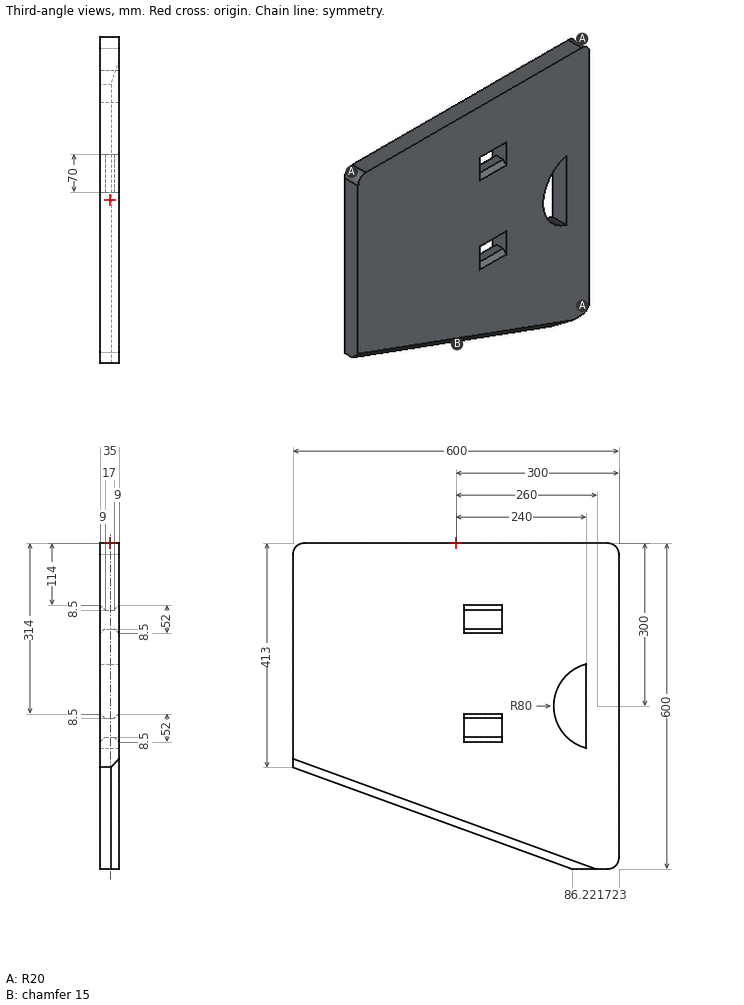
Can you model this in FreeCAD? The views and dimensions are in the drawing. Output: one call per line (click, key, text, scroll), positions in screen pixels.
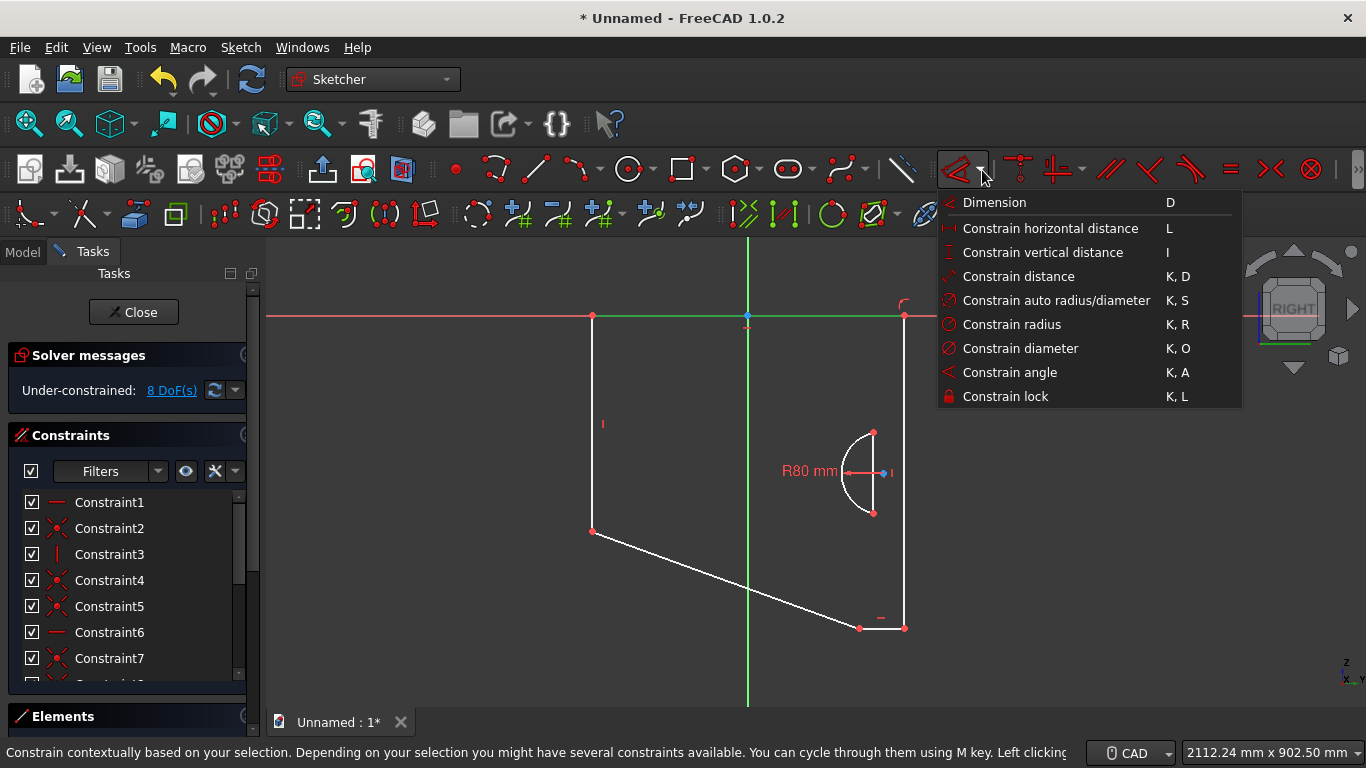
click(1090, 228)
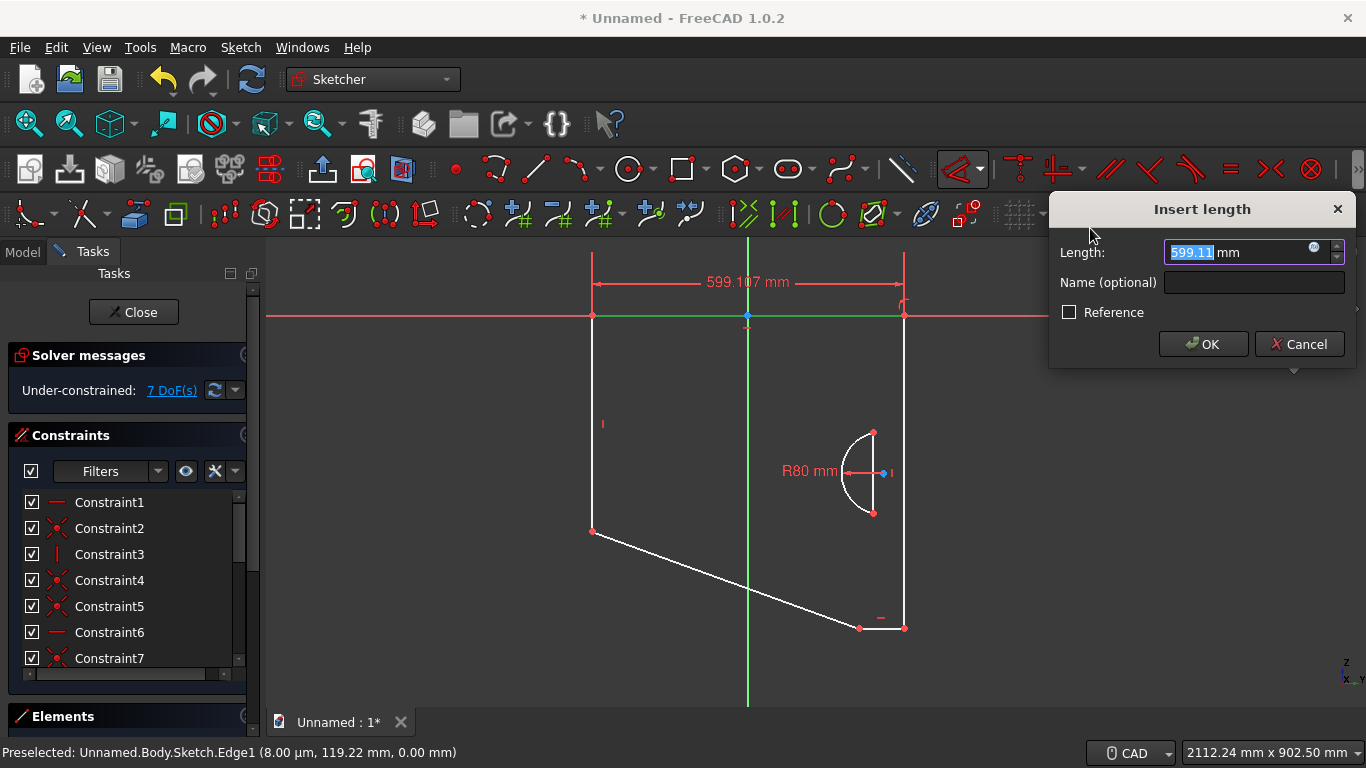
text(600)
key(Return)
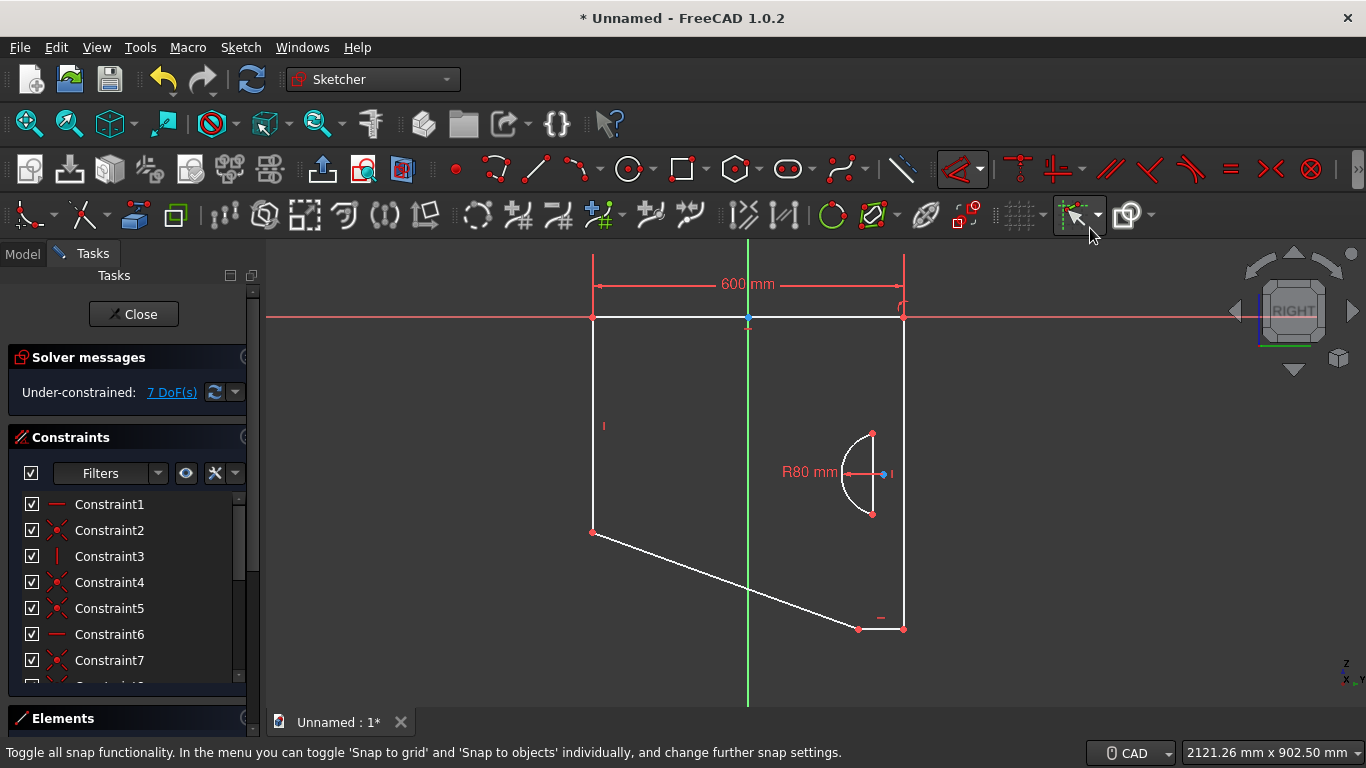
click(593, 382)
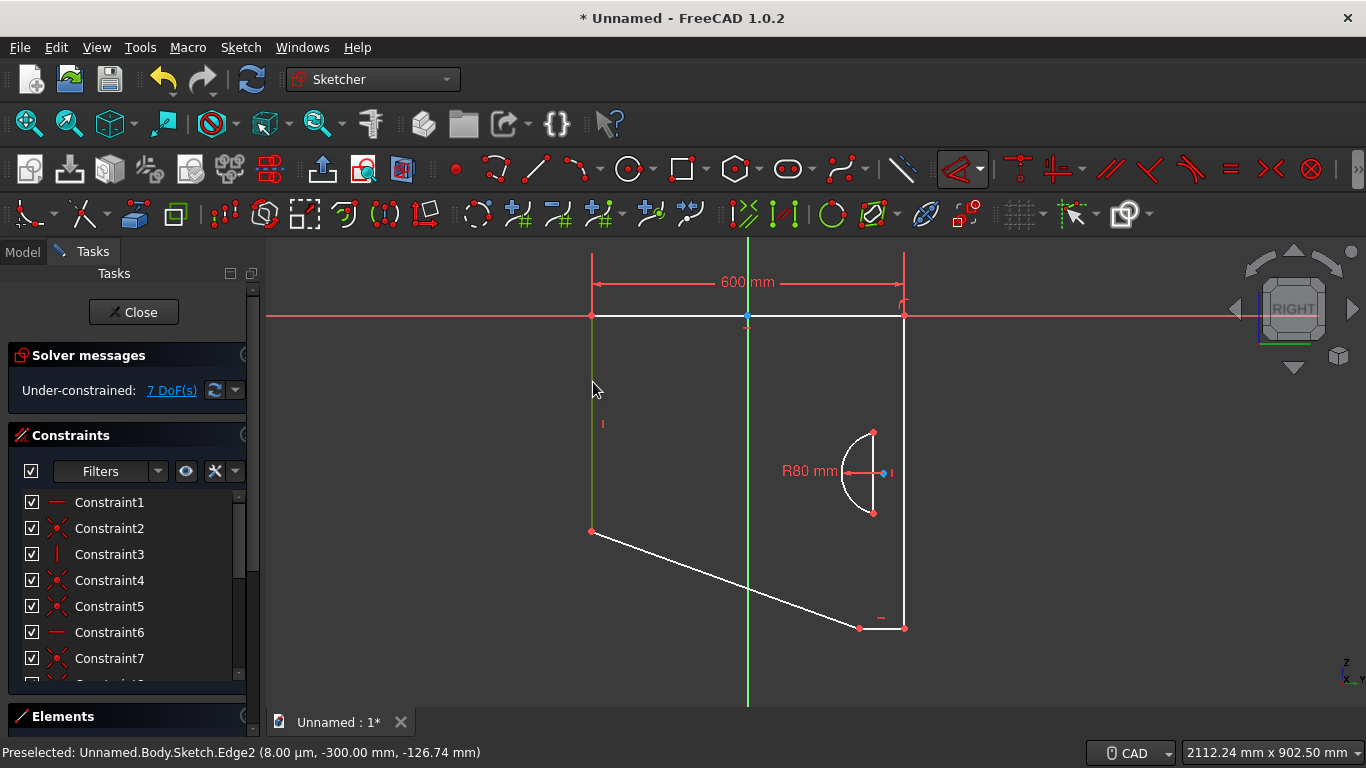
click(982, 170)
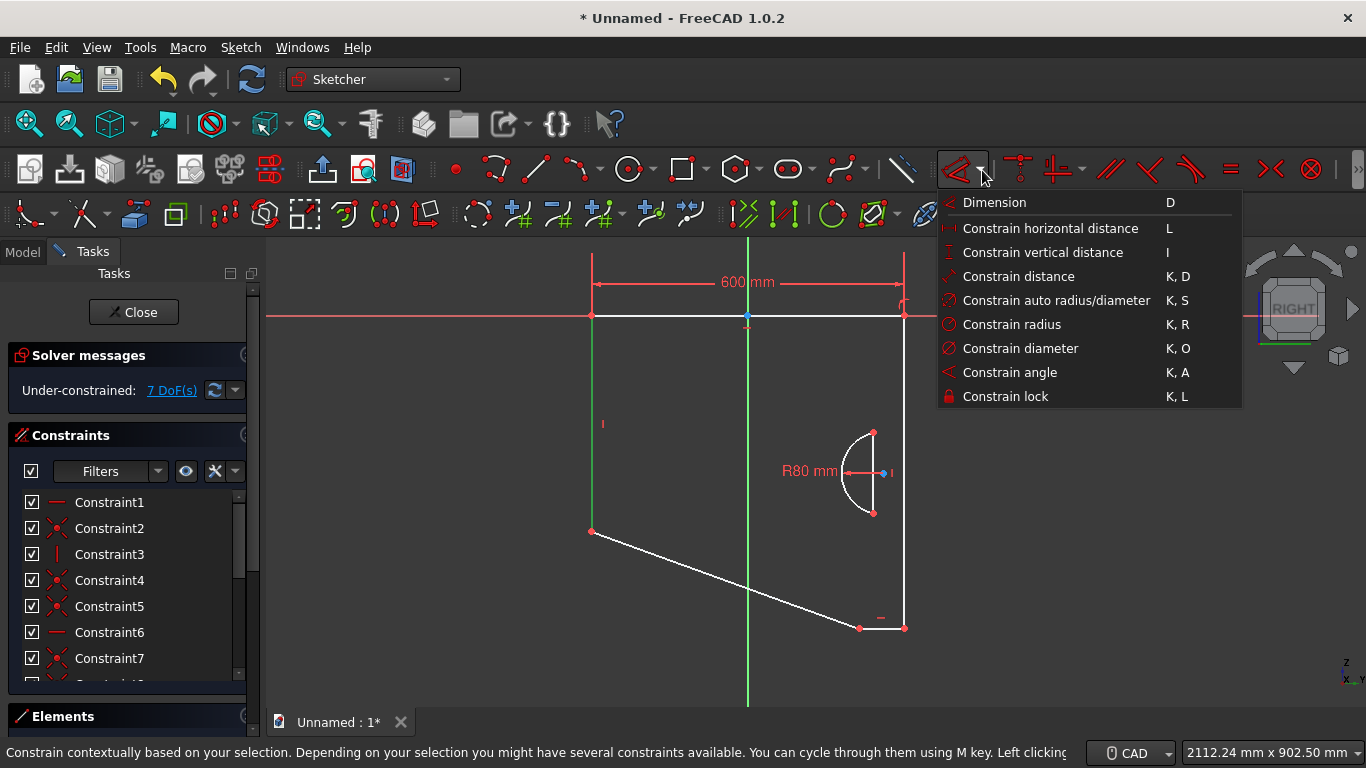
click(1090, 252)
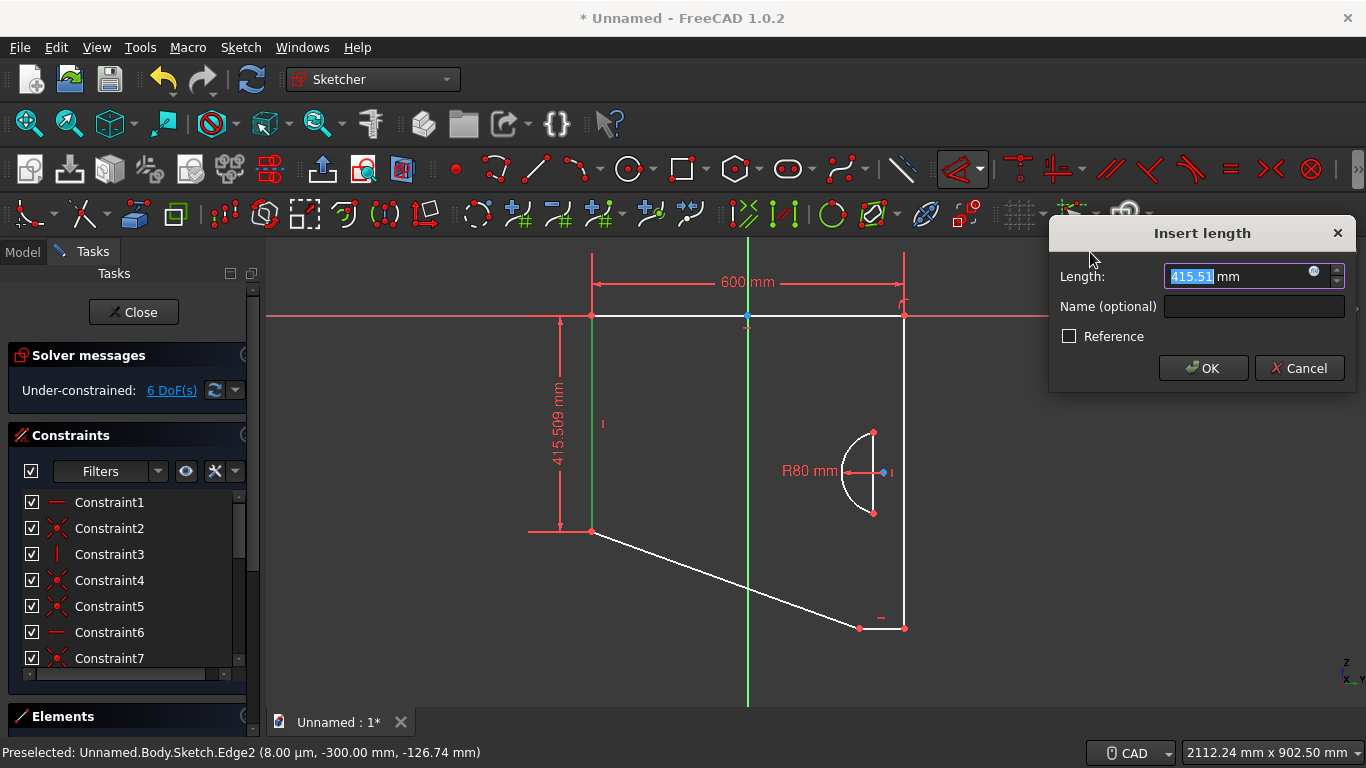
text(413)
key(Return)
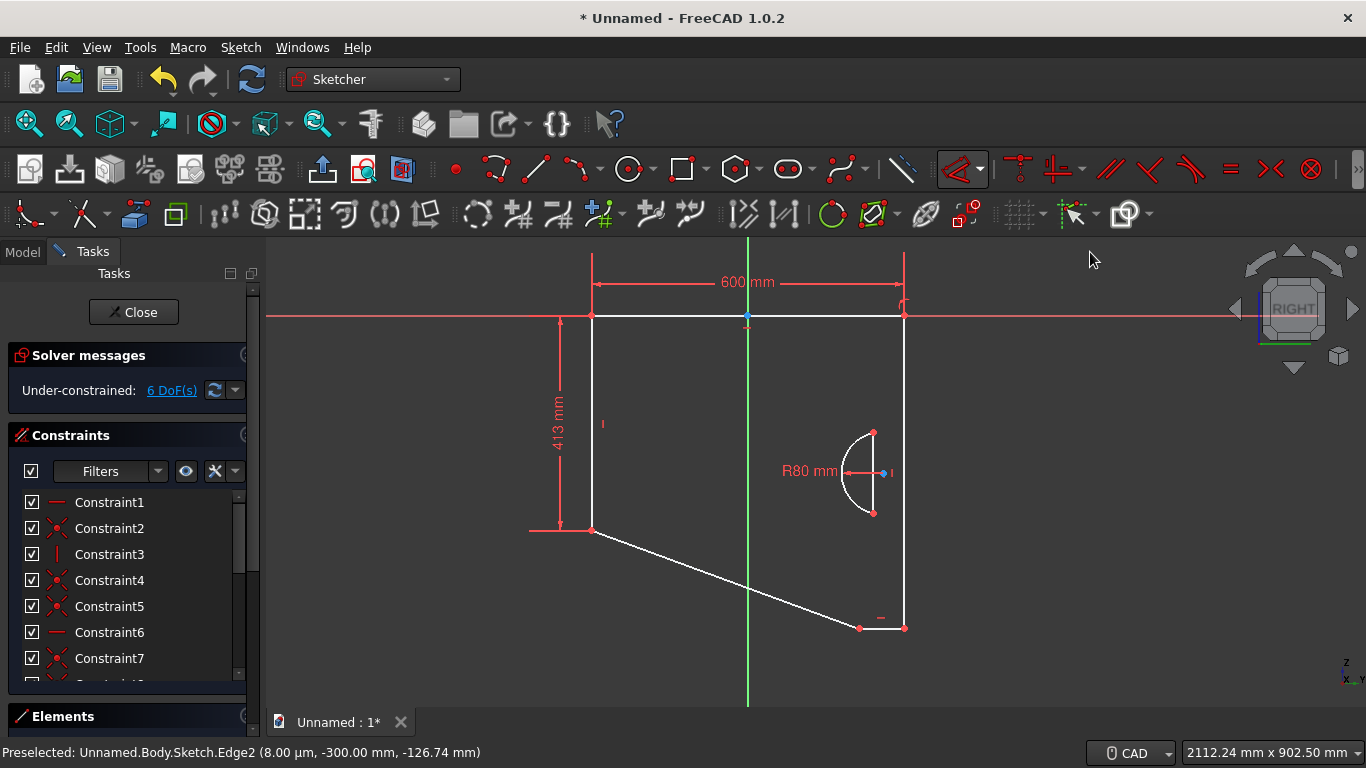
click(904, 535)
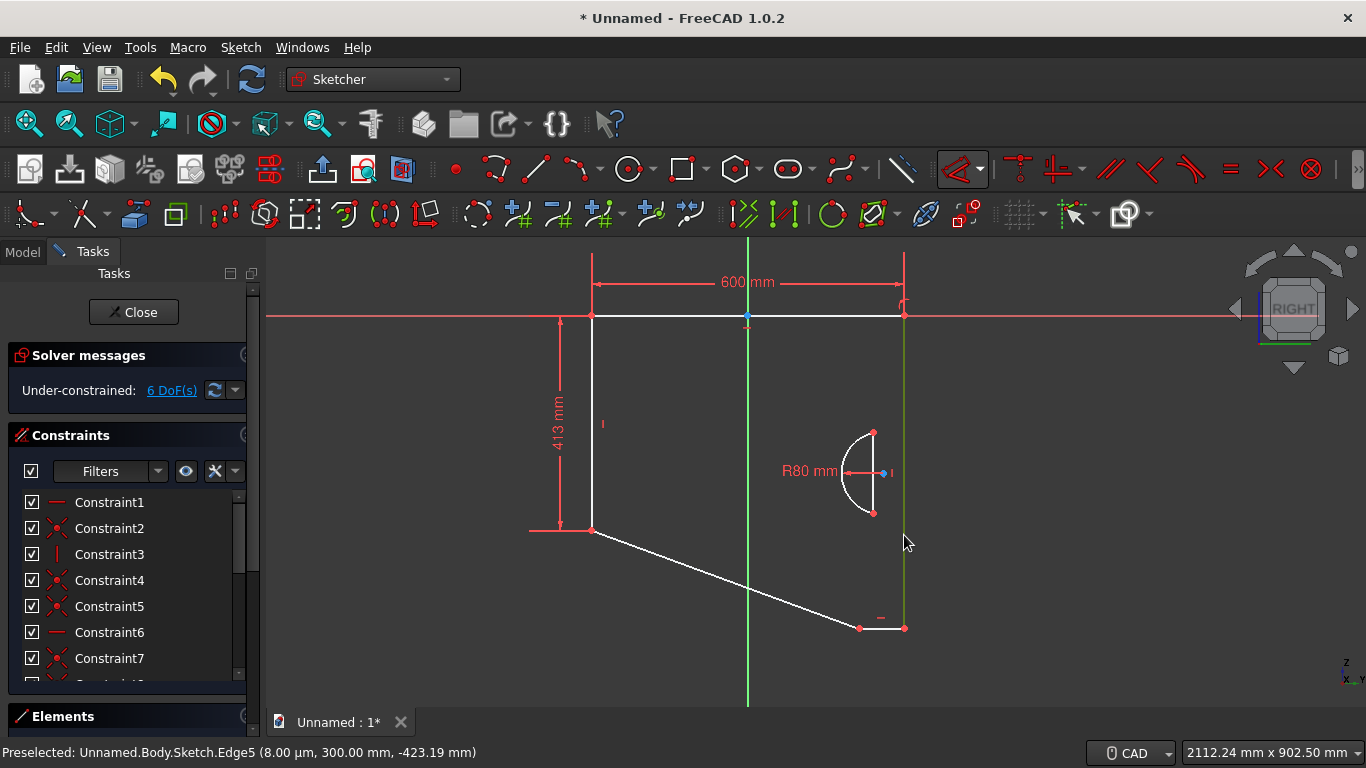
click(982, 170)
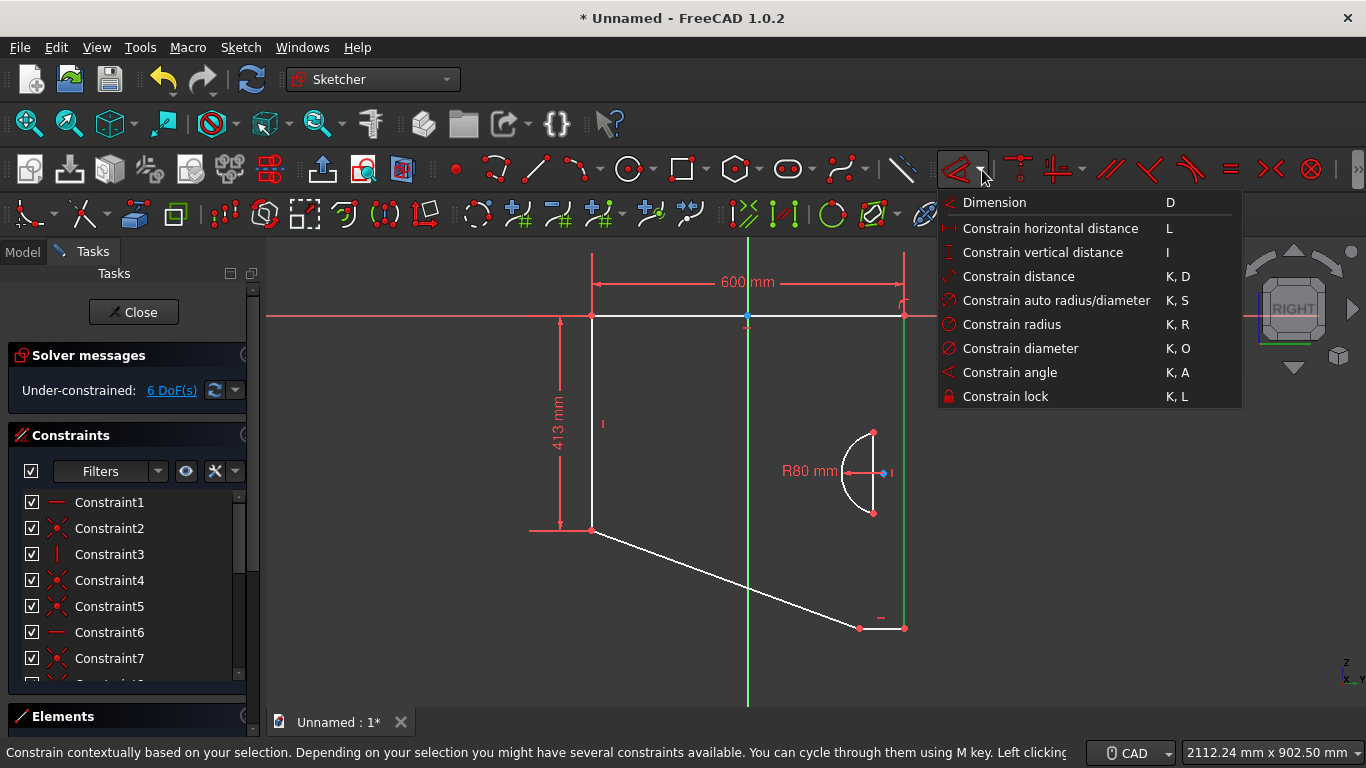
click(1090, 252)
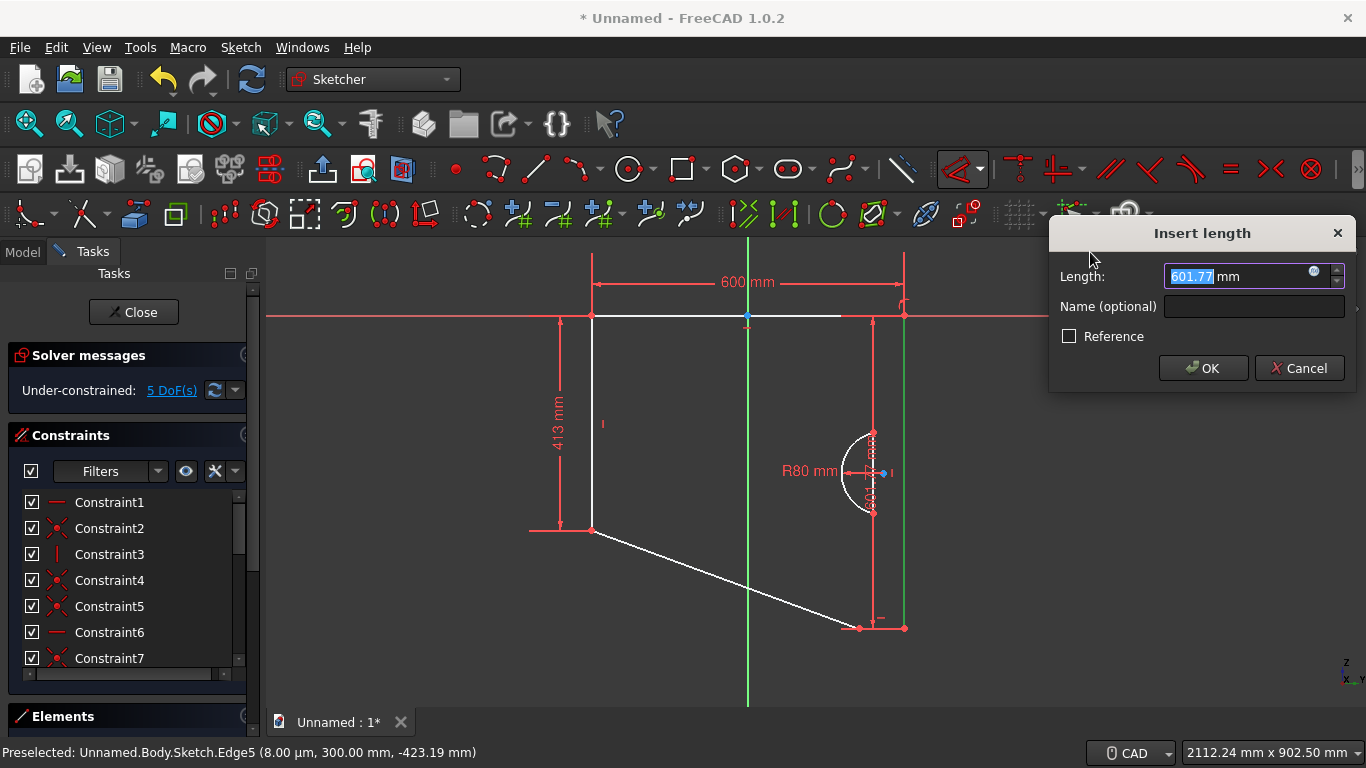
text(600)
key(Return)